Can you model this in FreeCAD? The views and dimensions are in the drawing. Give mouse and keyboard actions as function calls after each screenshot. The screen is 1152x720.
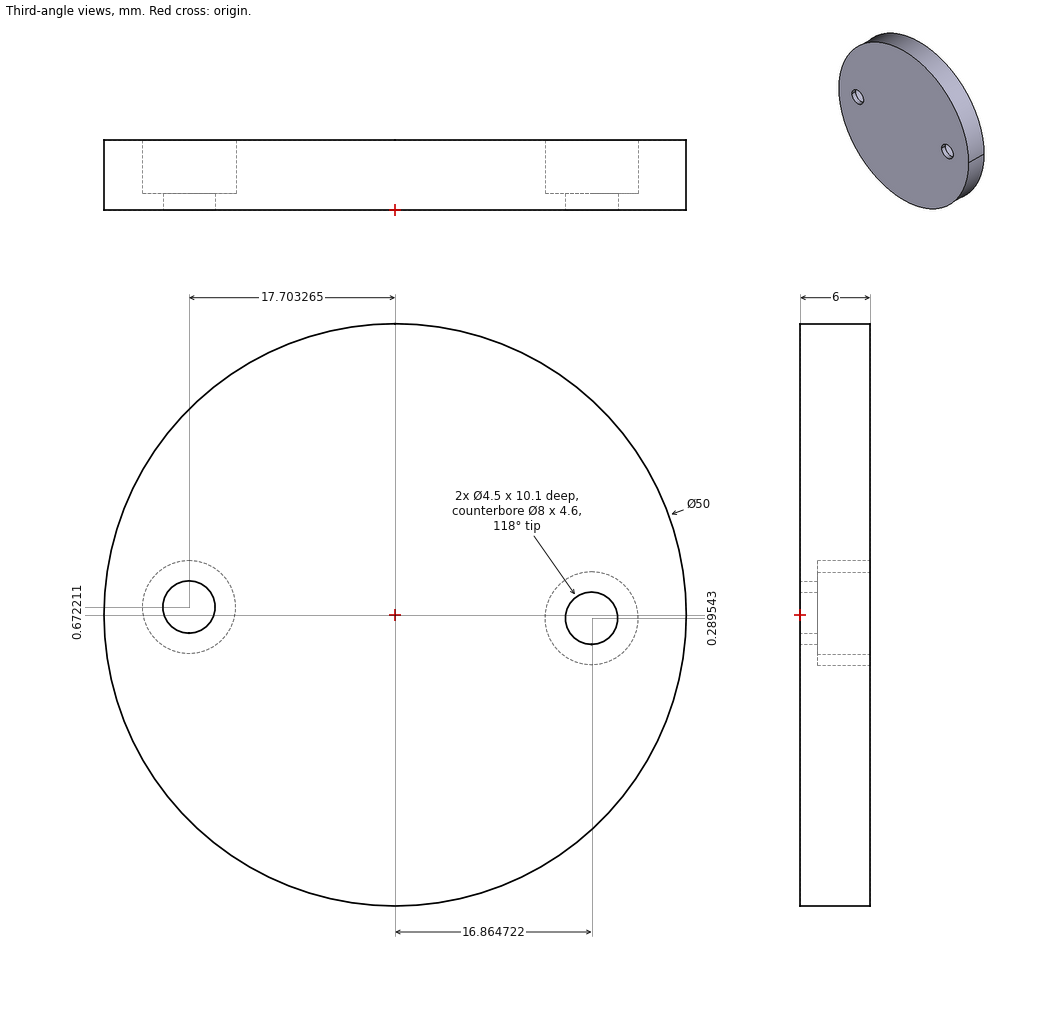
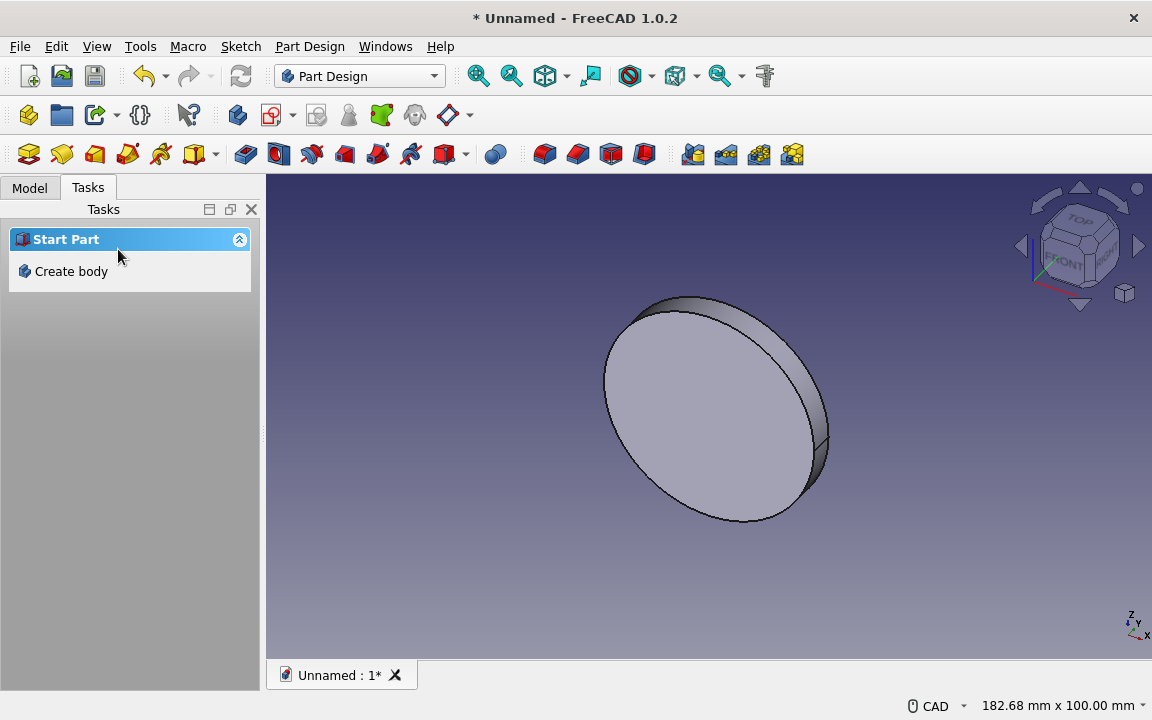
key(4)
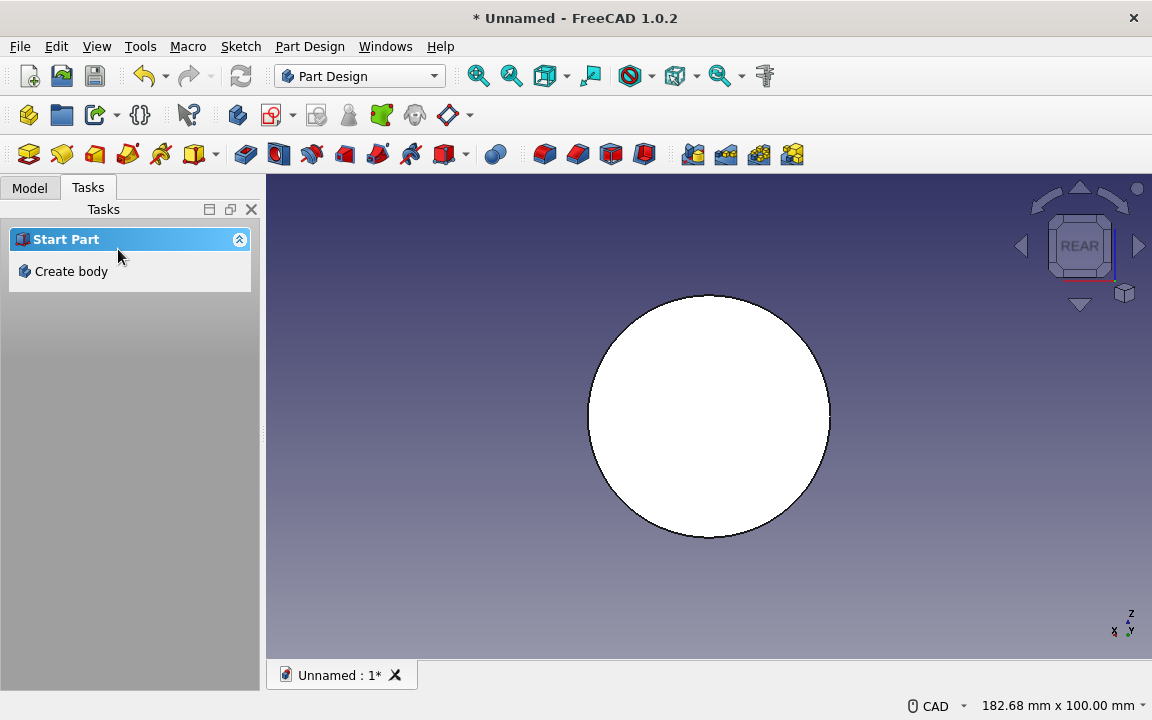
click(709, 415)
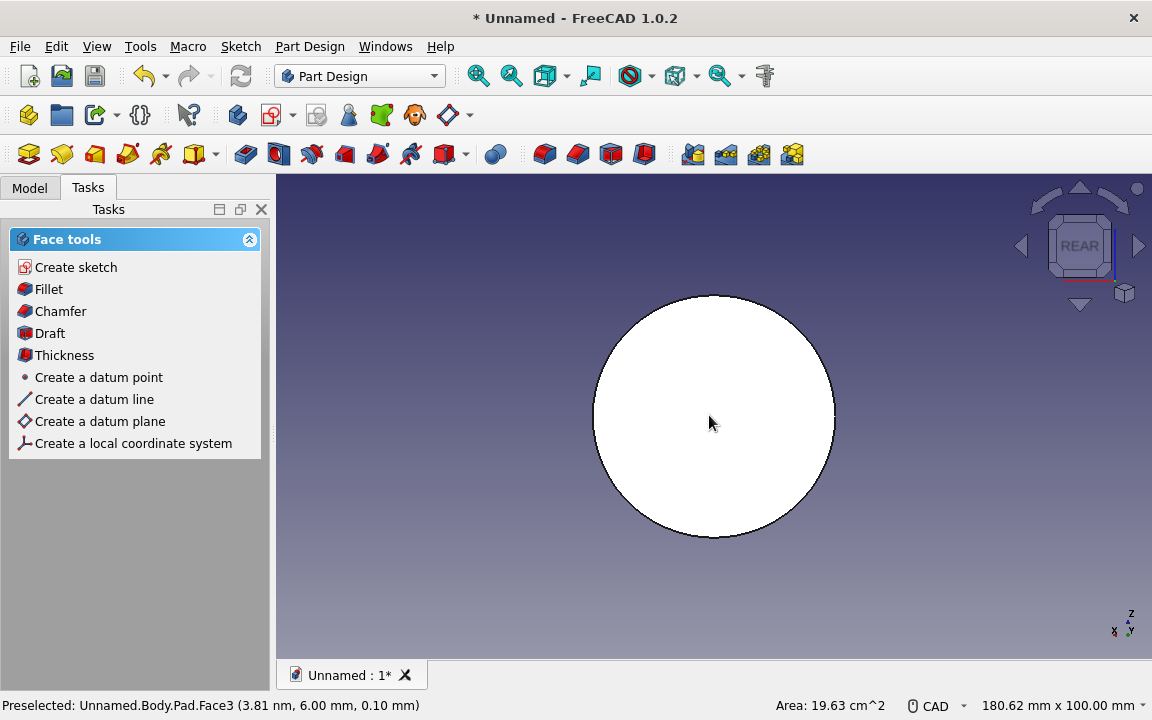
click(270, 116)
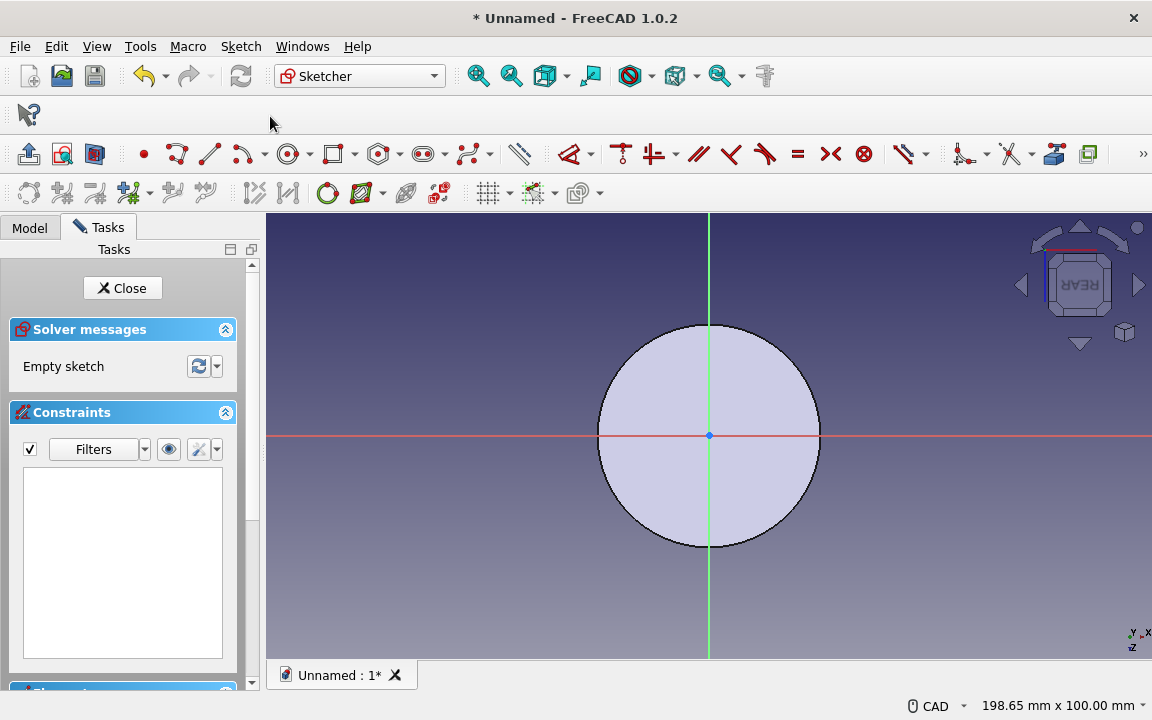
scroll(746, 437, up, 5)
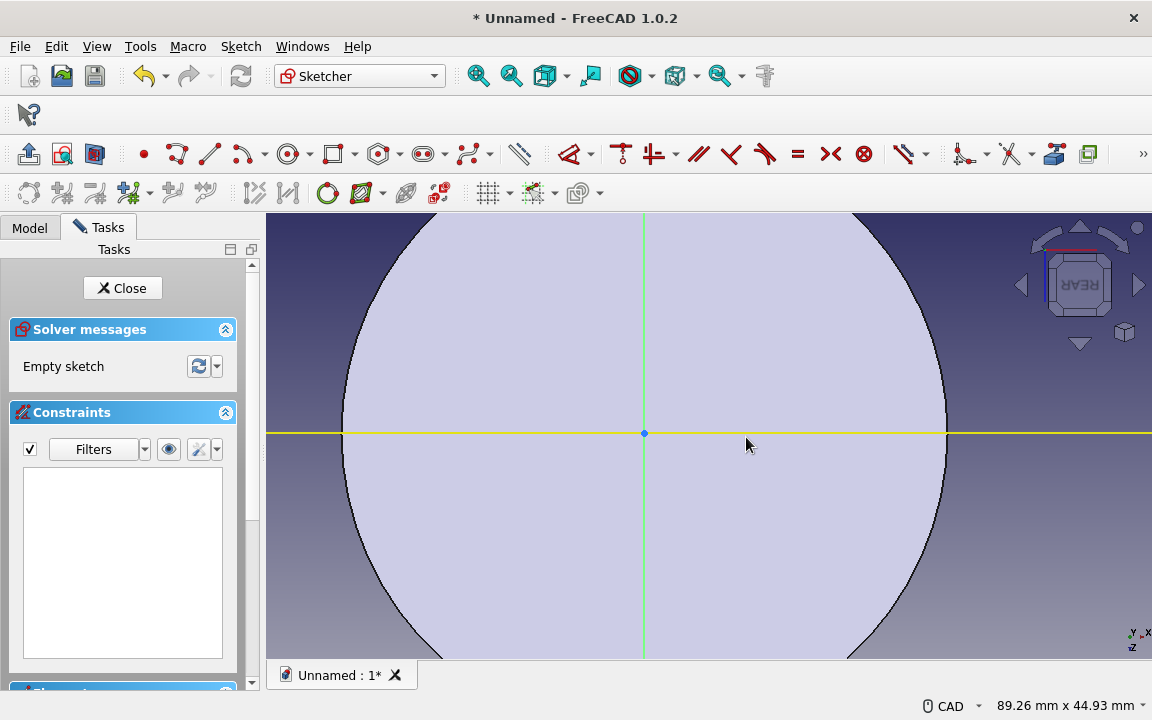
click(288, 154)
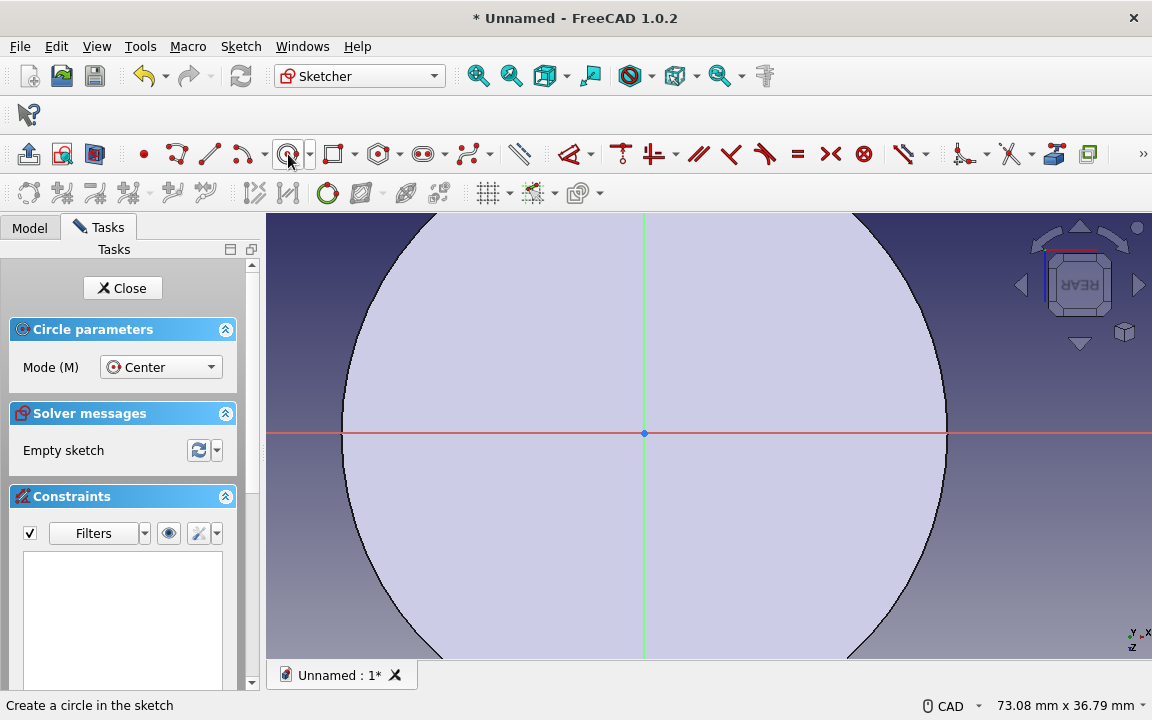
scroll(849, 430, up, 8)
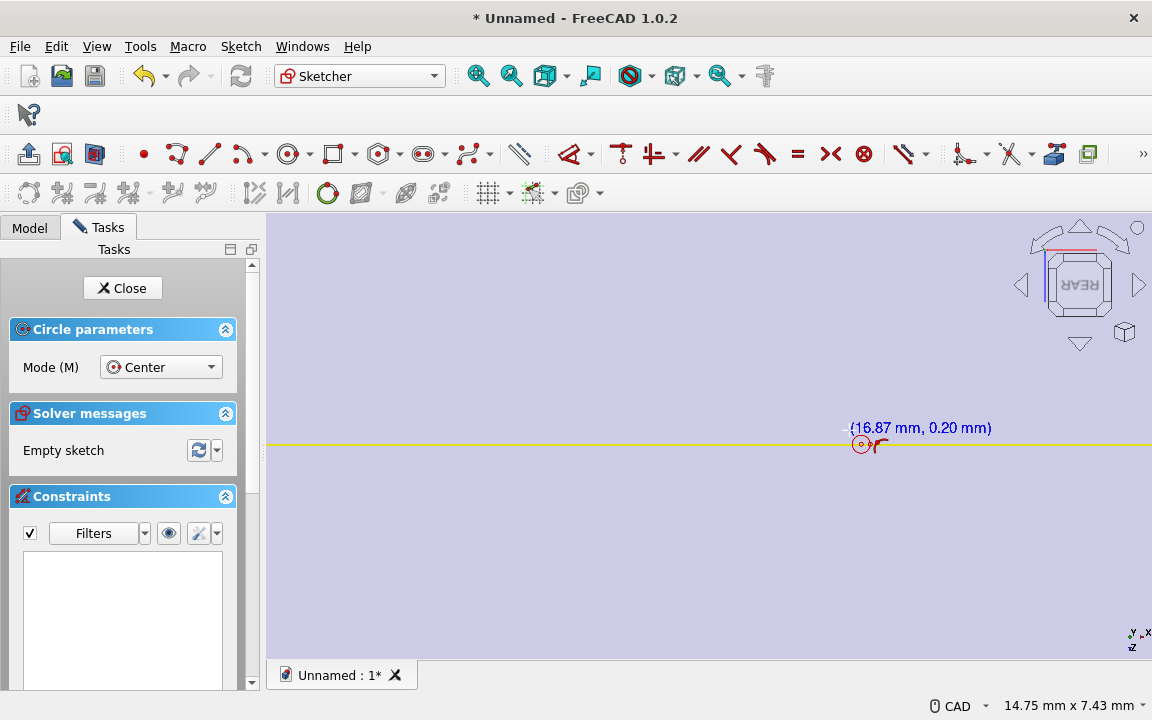
click(846, 428)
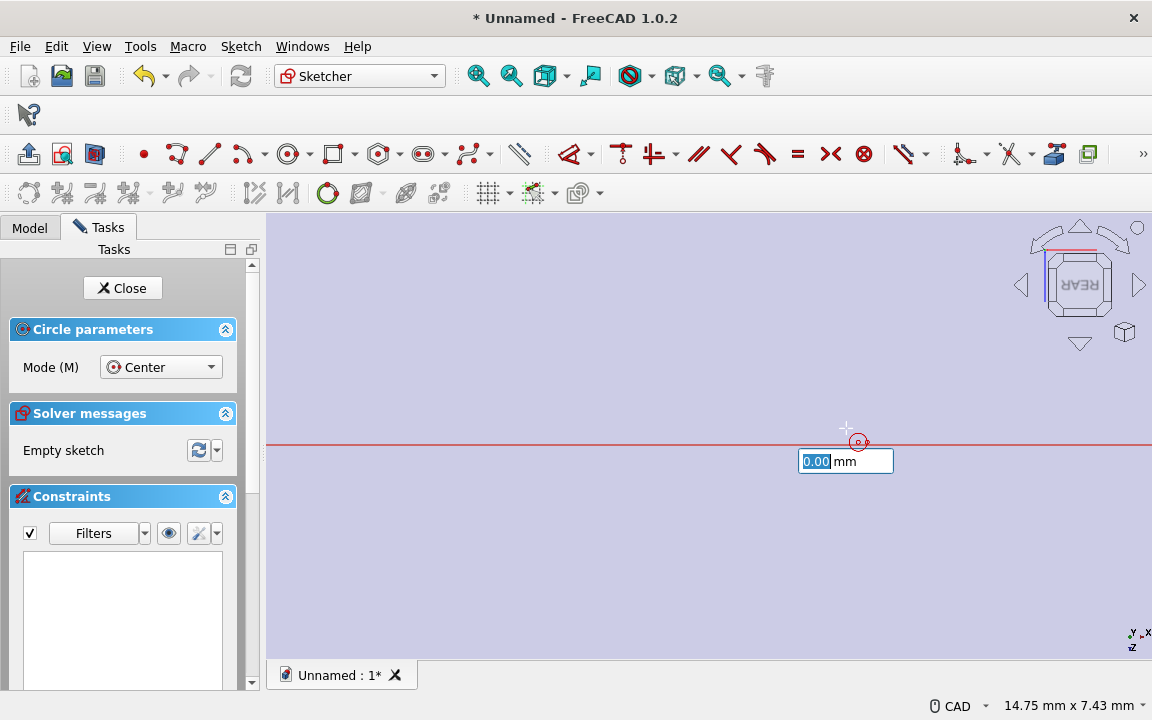
scroll(851, 431, down, 8)
move(870, 411)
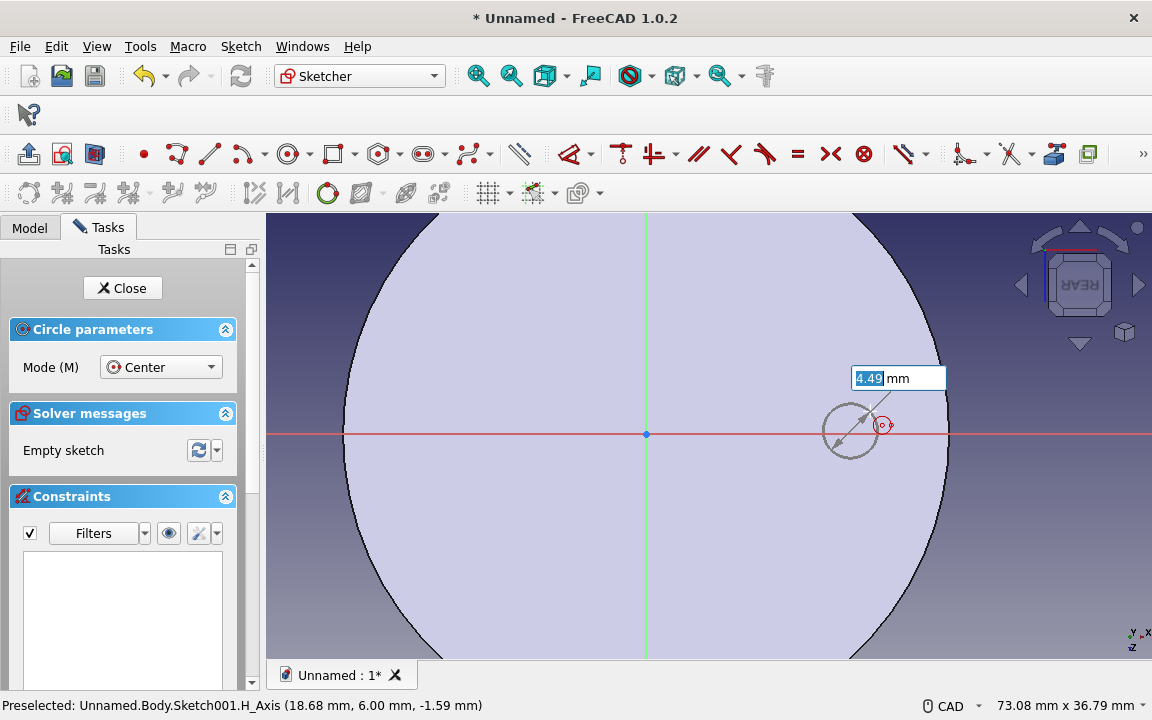
text(4.5)
key(Return)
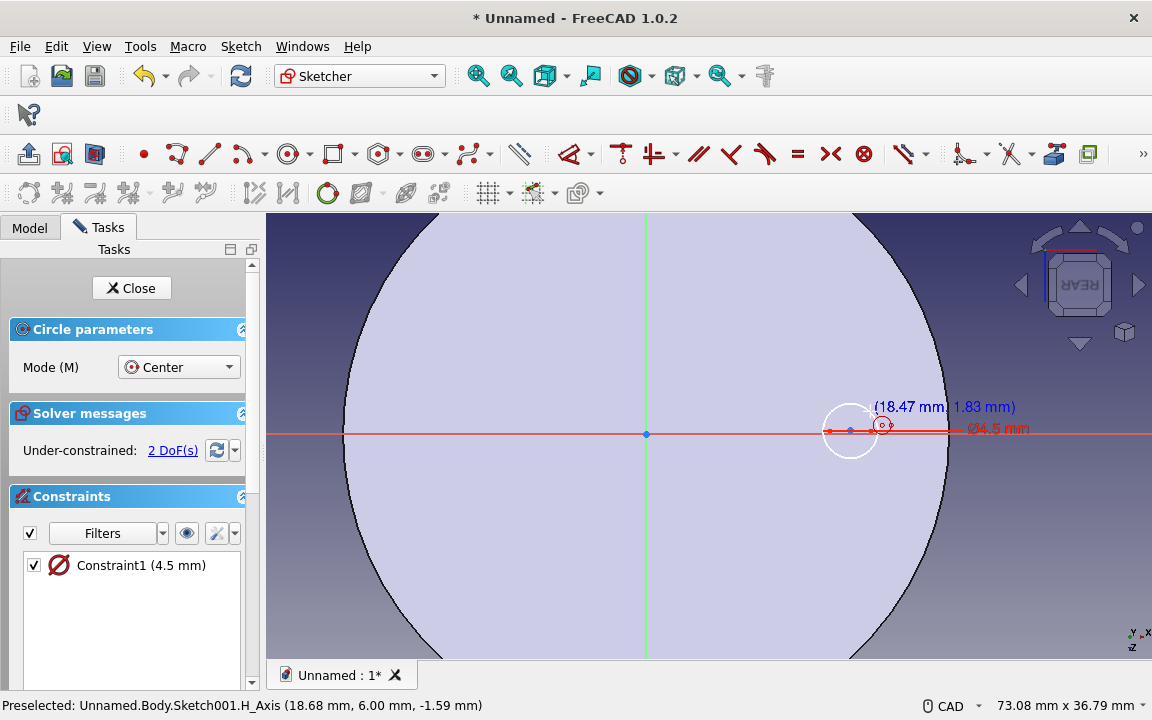
scroll(431, 442, up, 4)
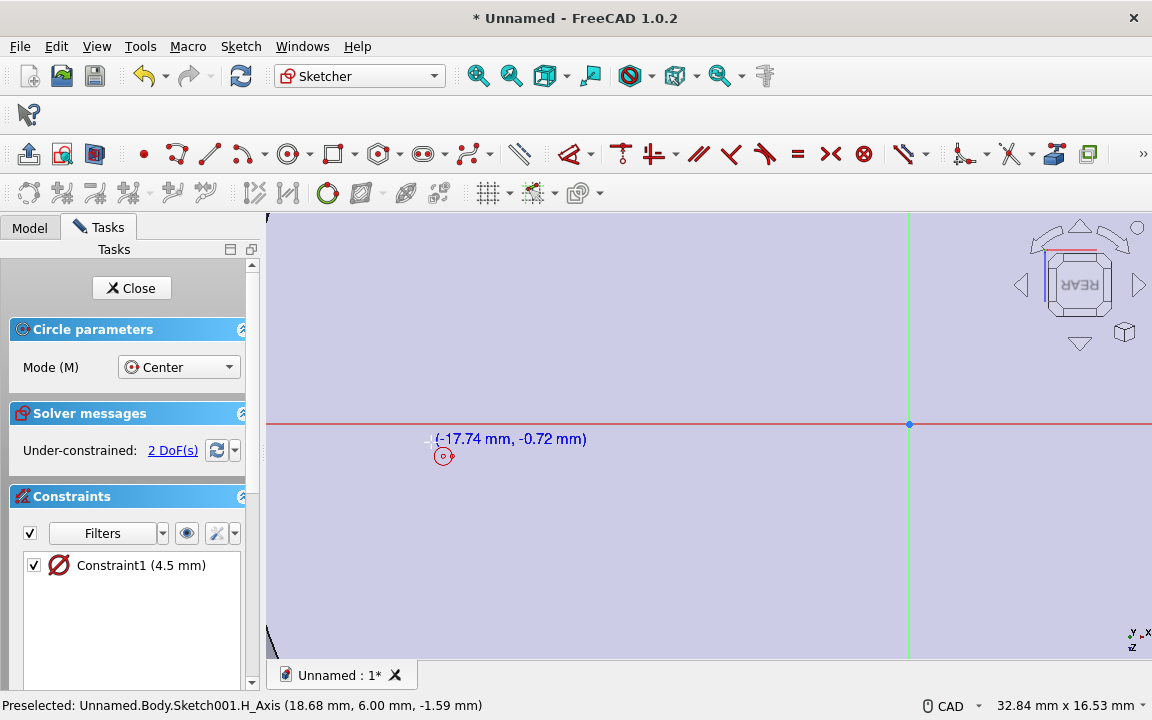
click(432, 442)
move(475, 399)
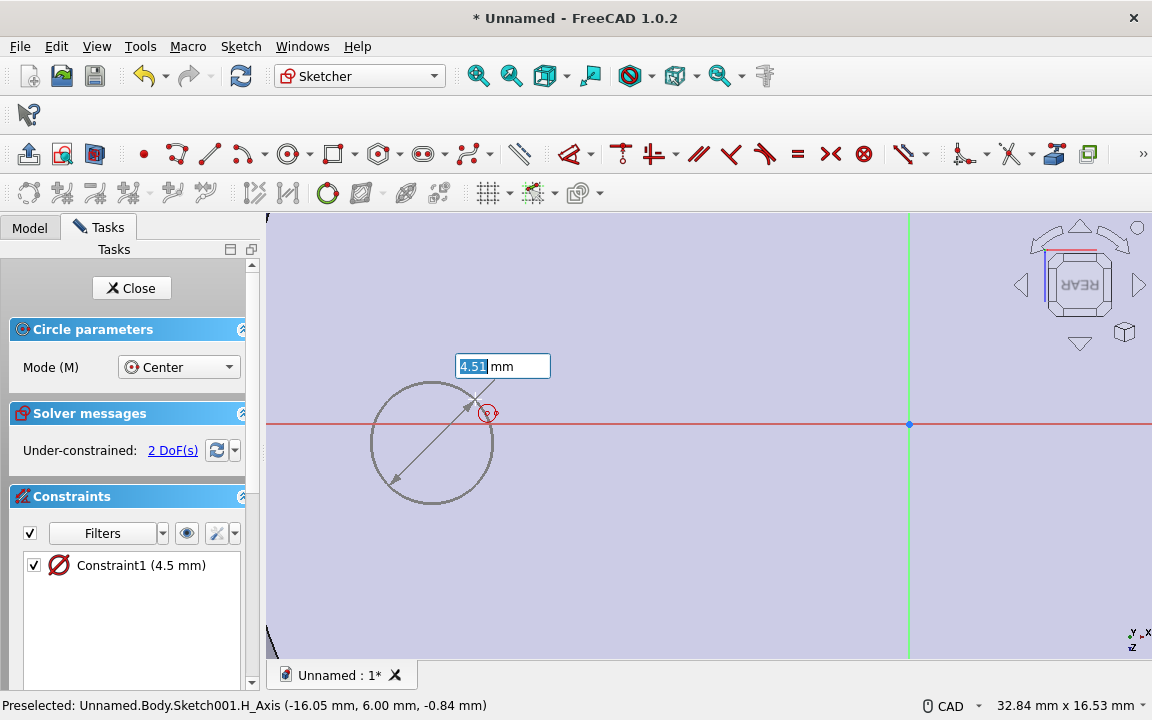
text(4.5)
key(Return)
key(Escape)